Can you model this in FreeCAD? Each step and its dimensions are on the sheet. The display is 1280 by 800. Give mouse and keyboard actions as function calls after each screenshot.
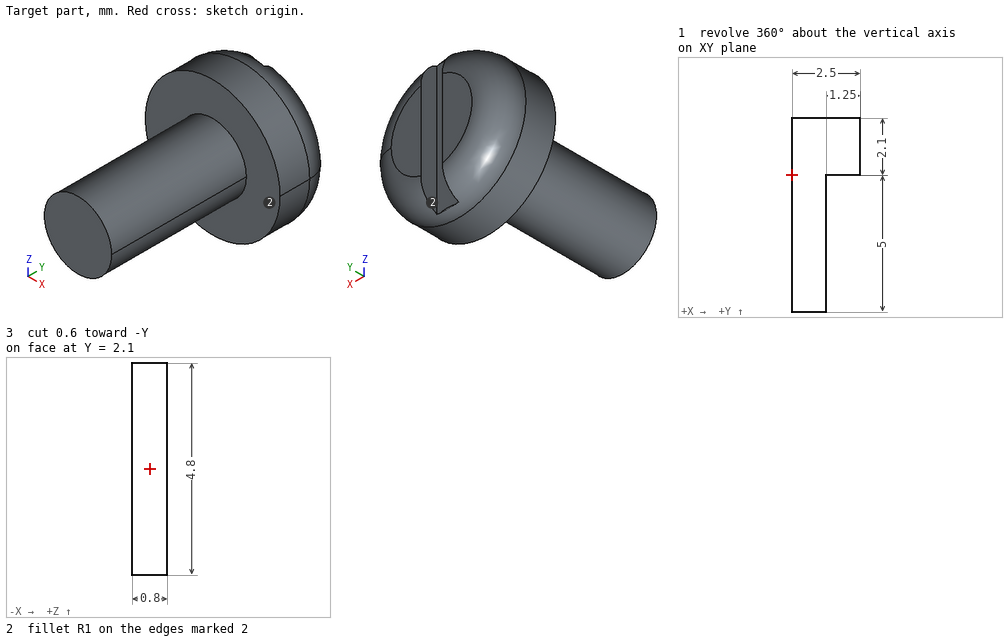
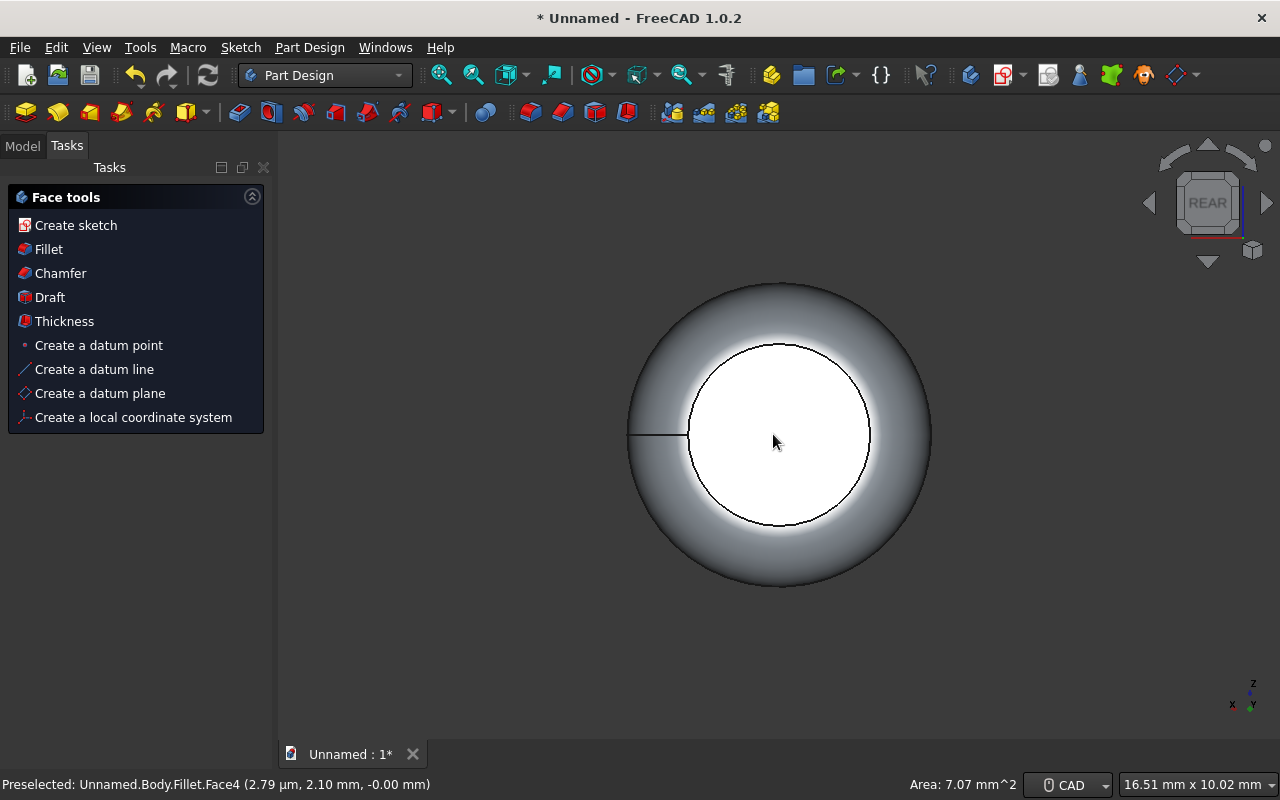
click(1004, 76)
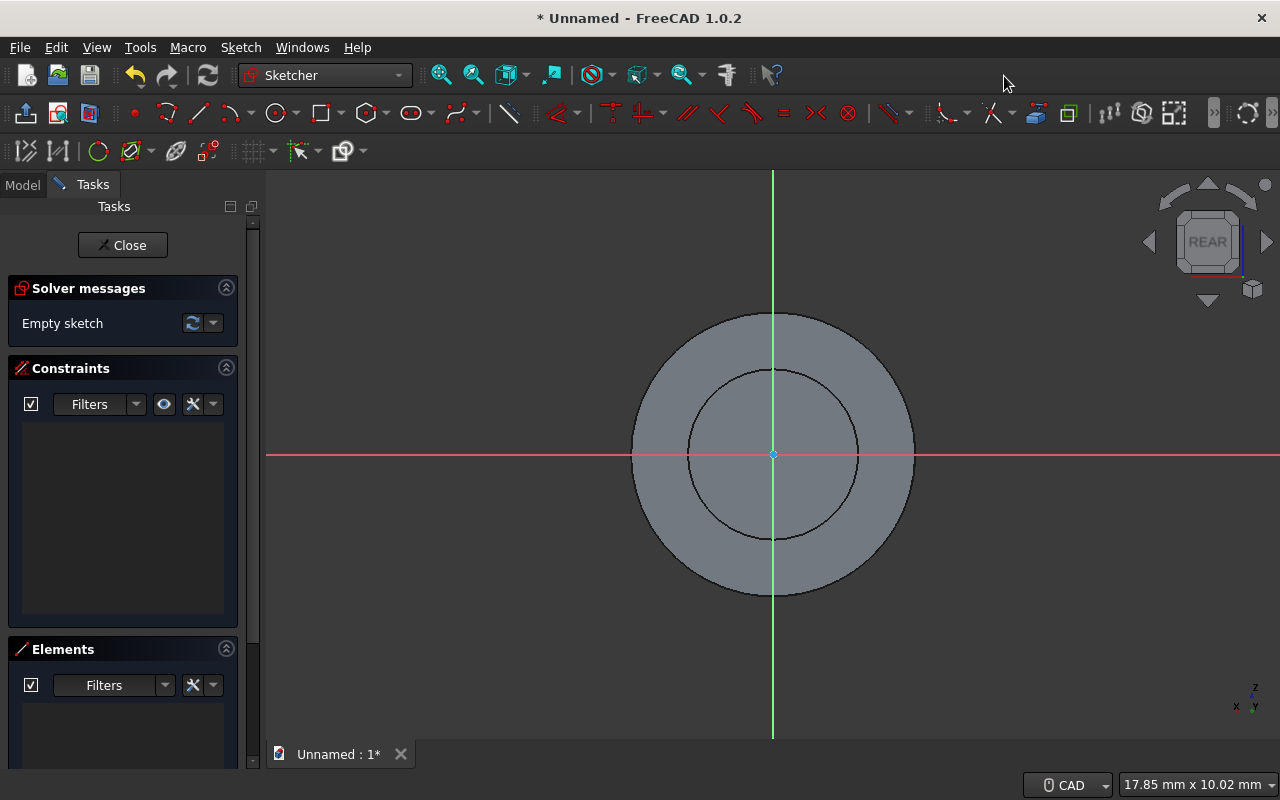
click(344, 114)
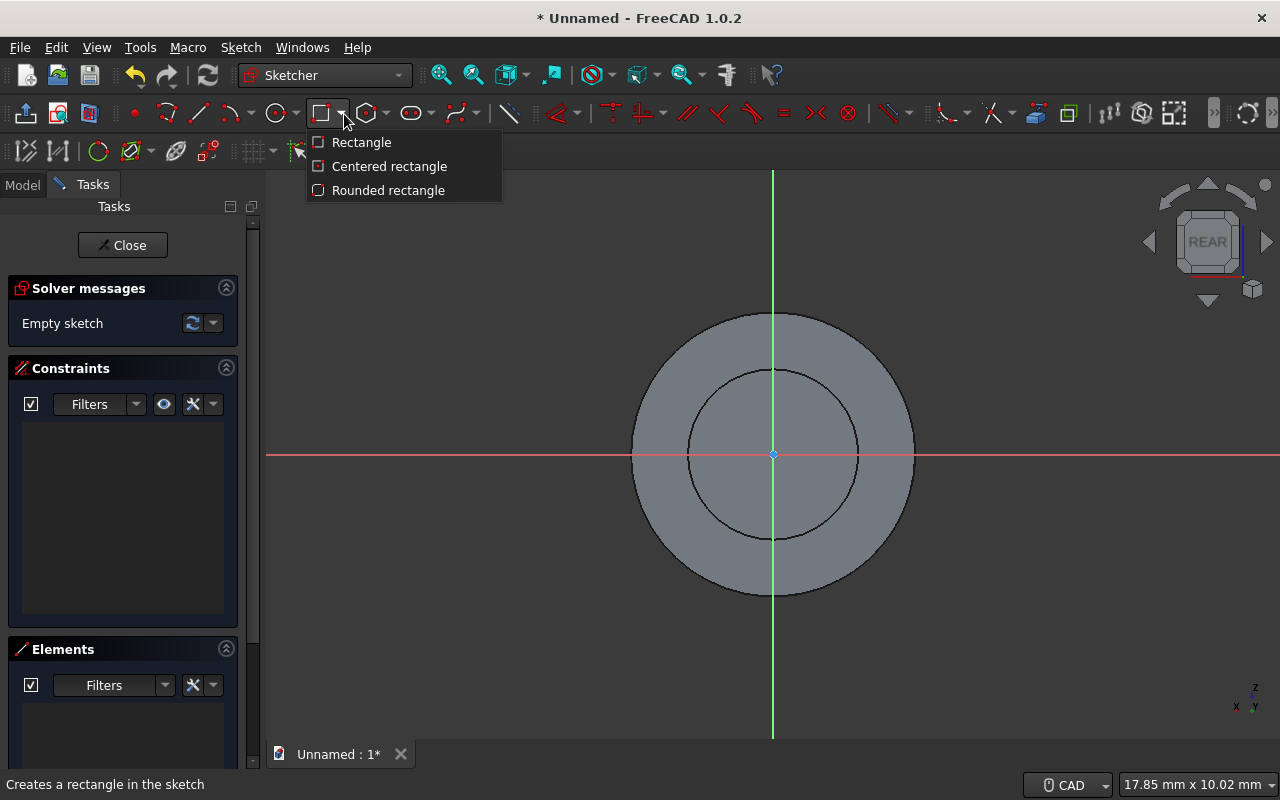
click(404, 166)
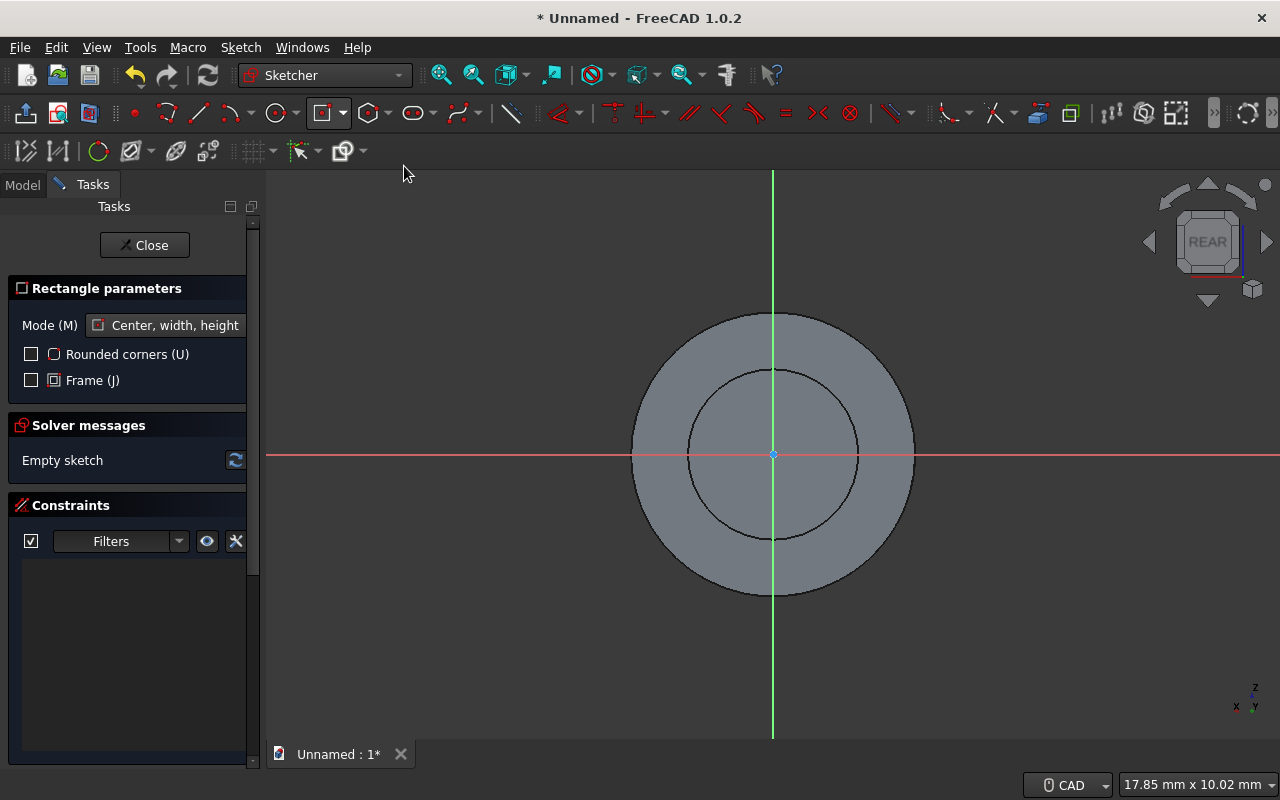
click(773, 454)
click(796, 318)
key(Escape)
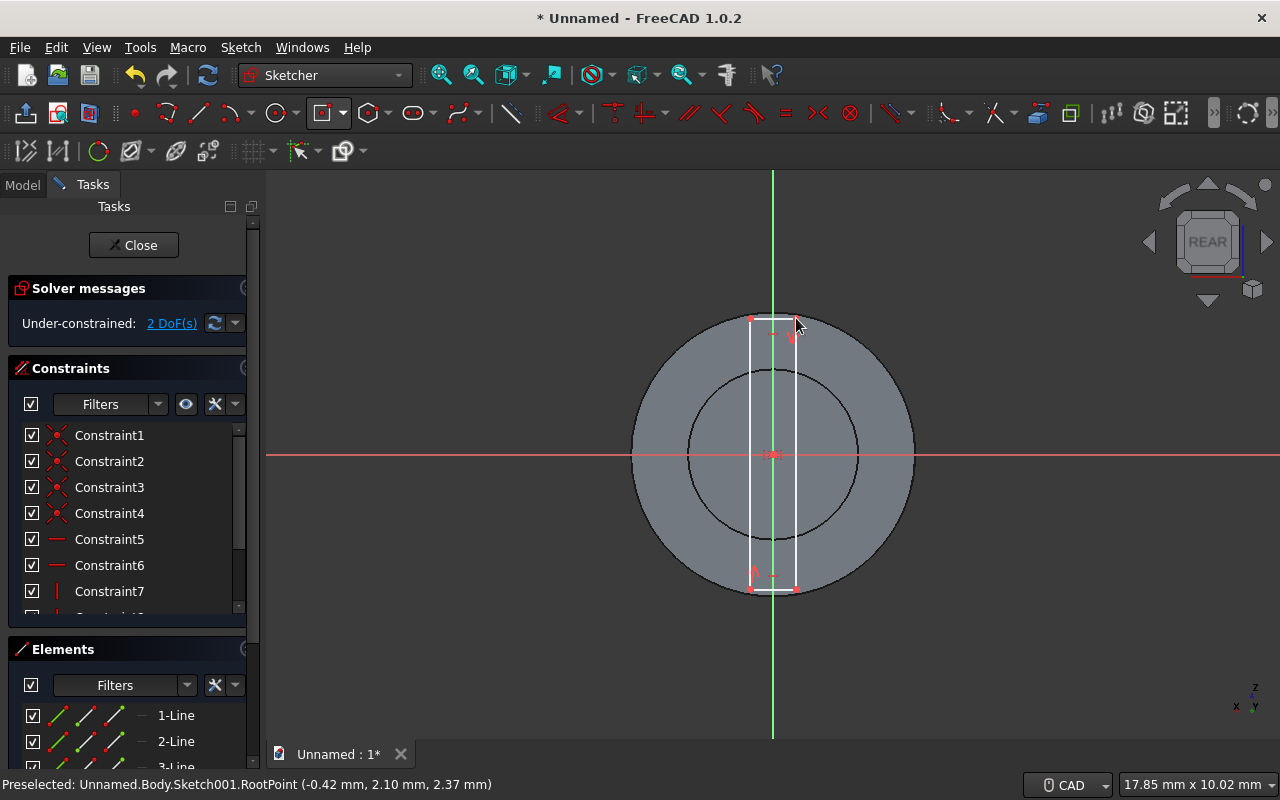
click(558, 114)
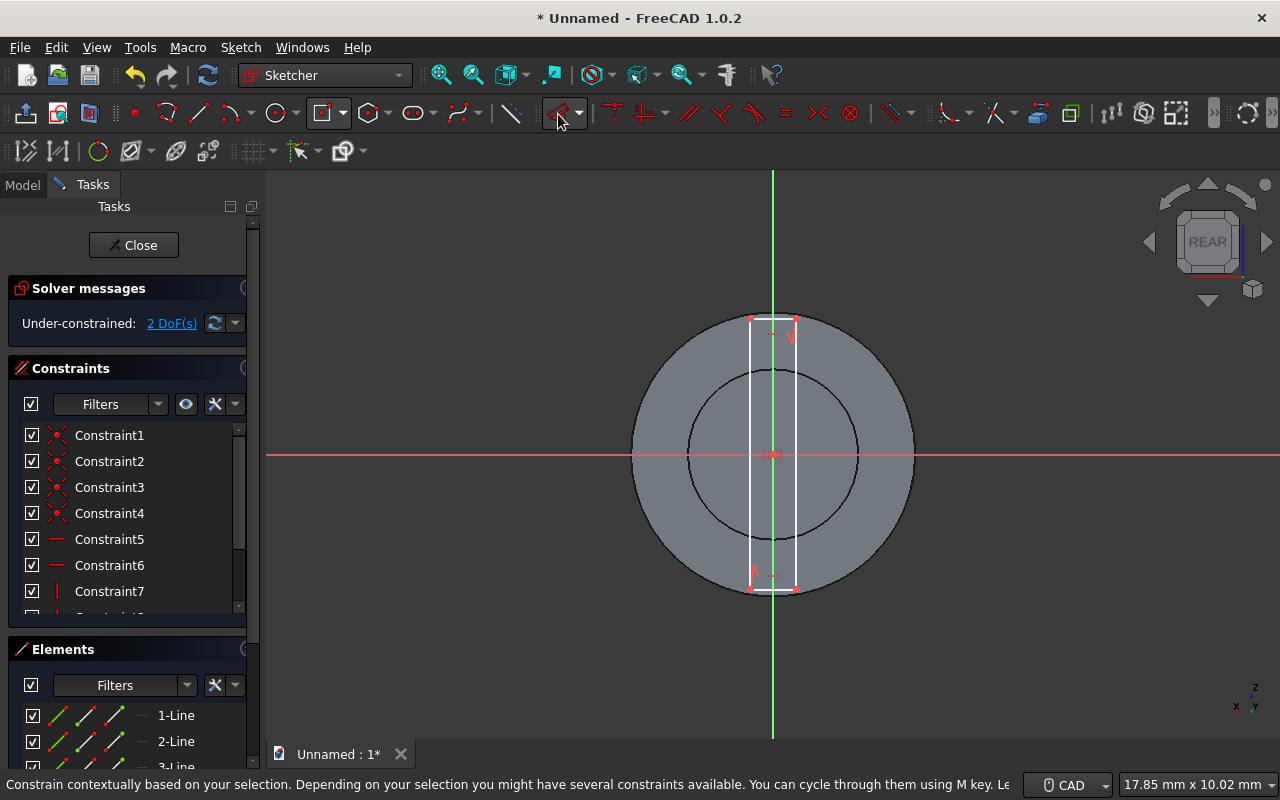
scroll(764, 590, up, 3)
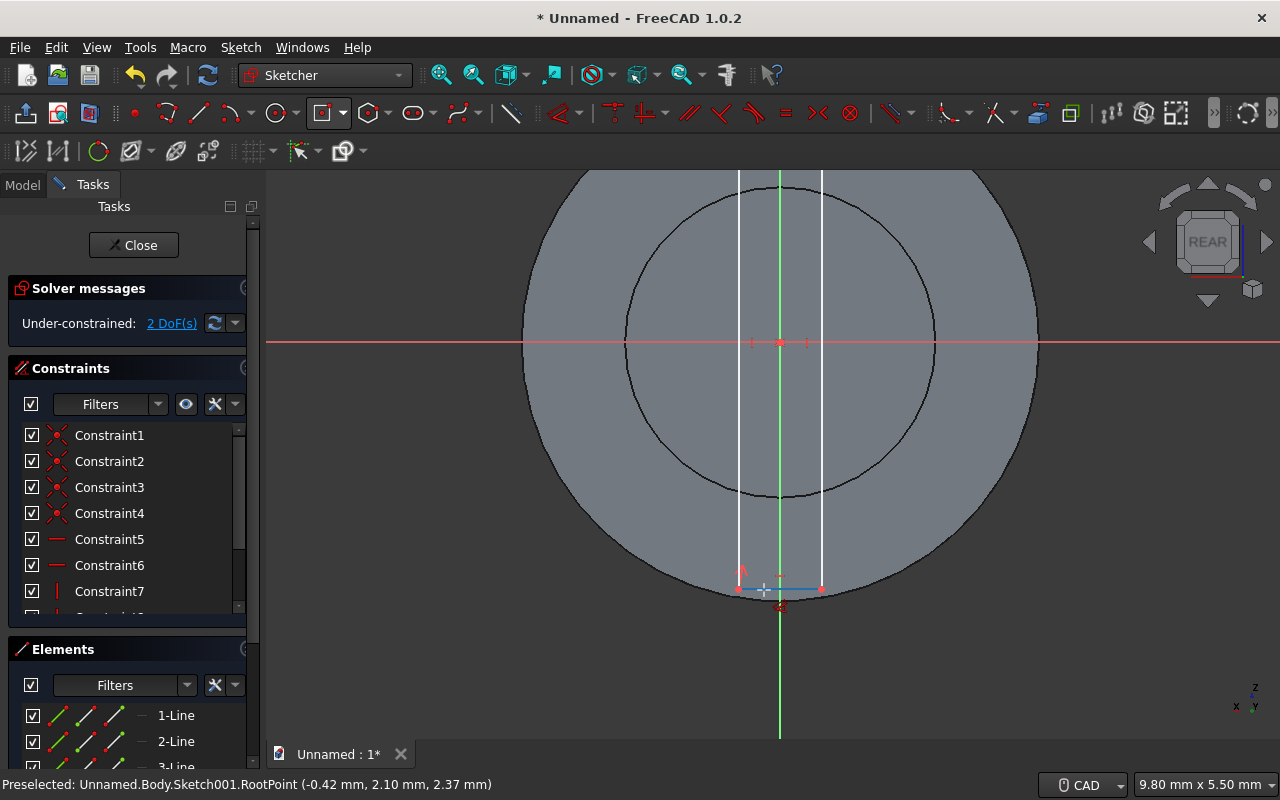
click(764, 589)
click(761, 623)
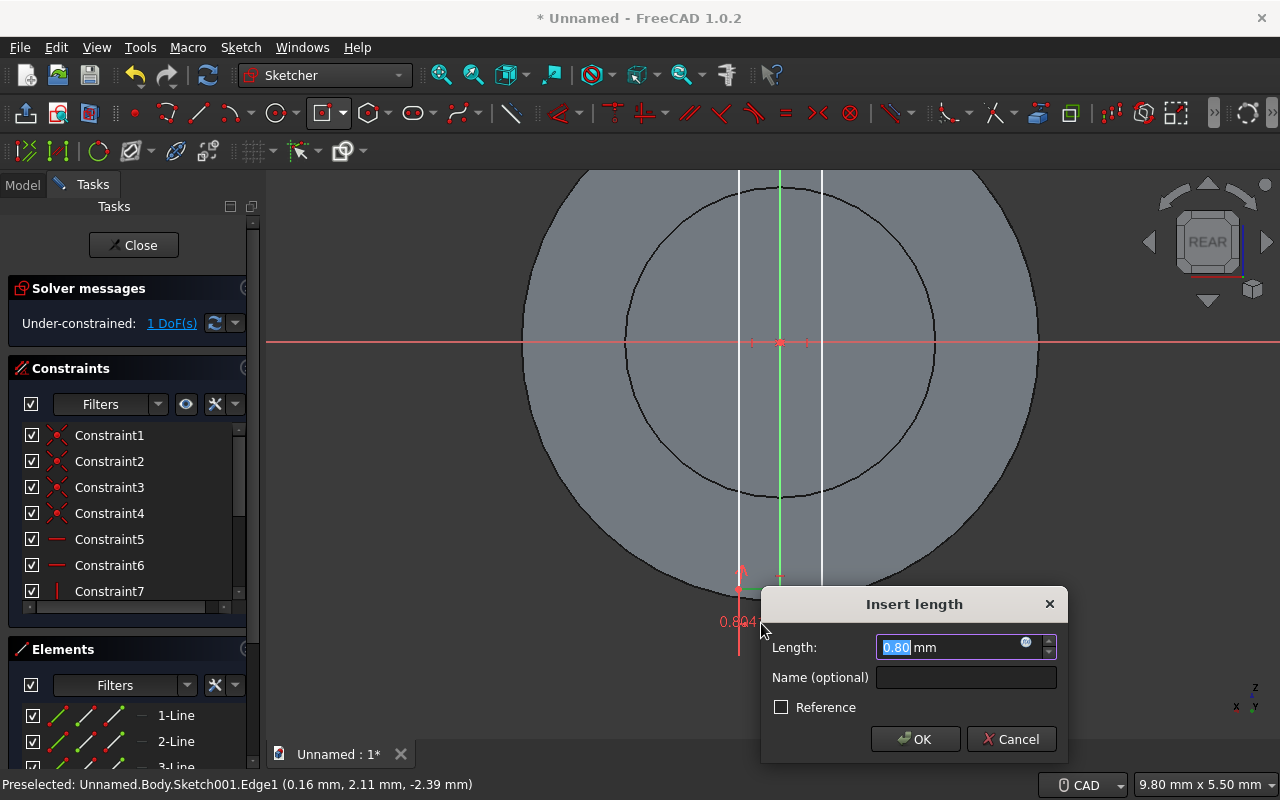
text(0.8)
key(Return)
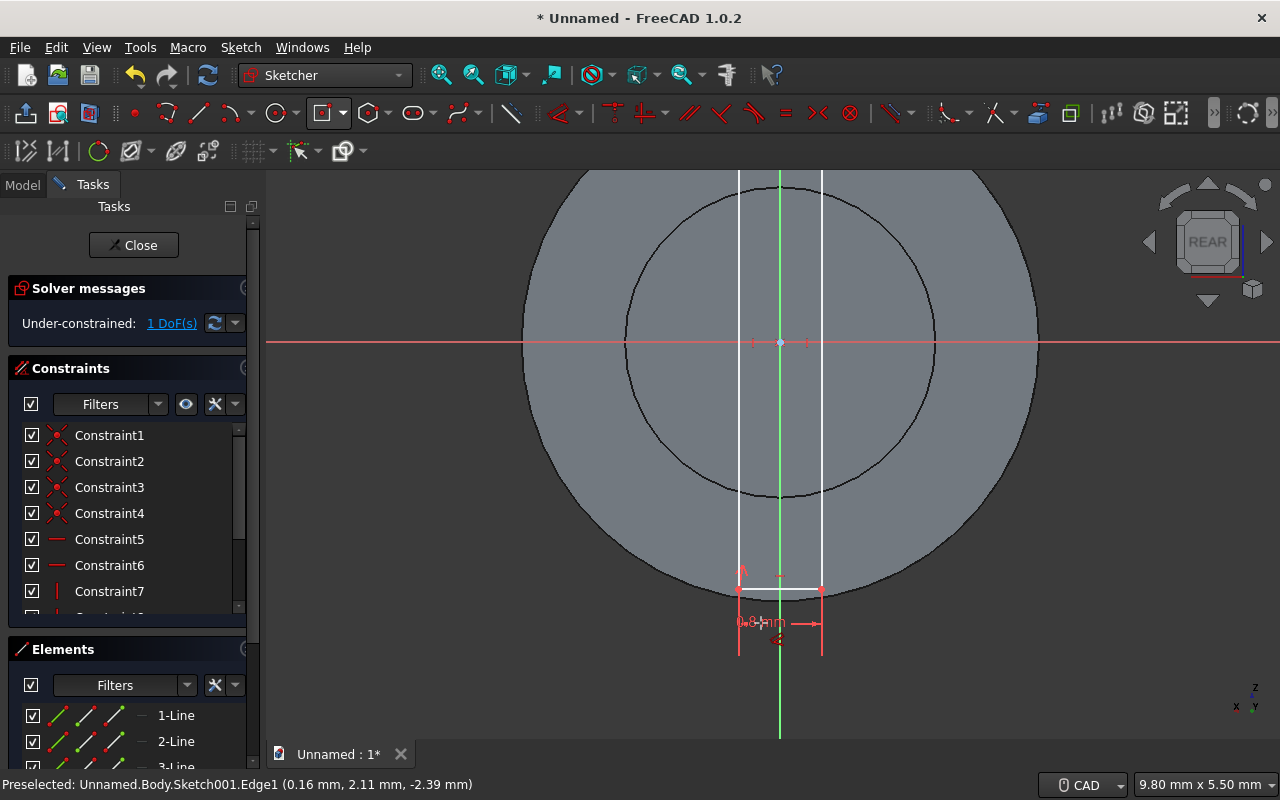
click(822, 441)
click(856, 394)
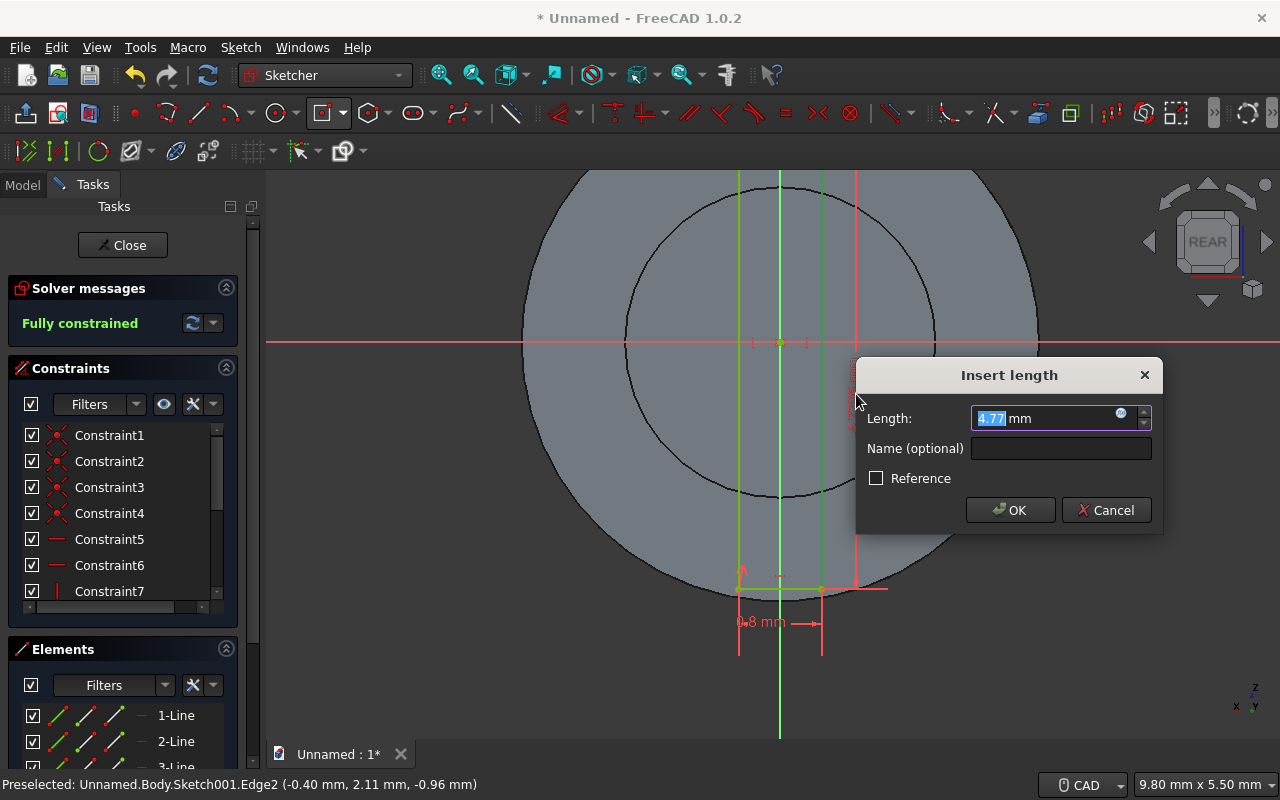
text(4.8)
key(Return)
key(Escape)